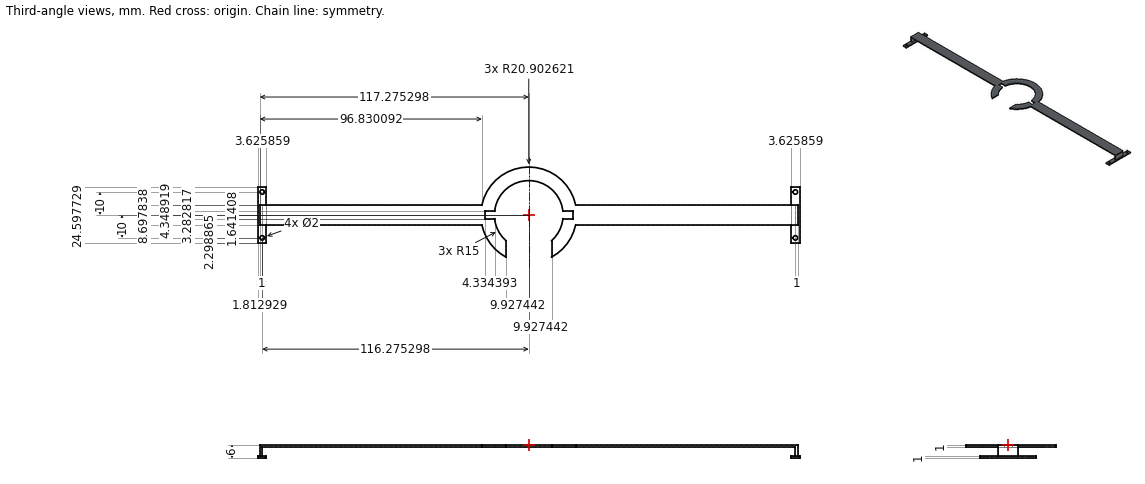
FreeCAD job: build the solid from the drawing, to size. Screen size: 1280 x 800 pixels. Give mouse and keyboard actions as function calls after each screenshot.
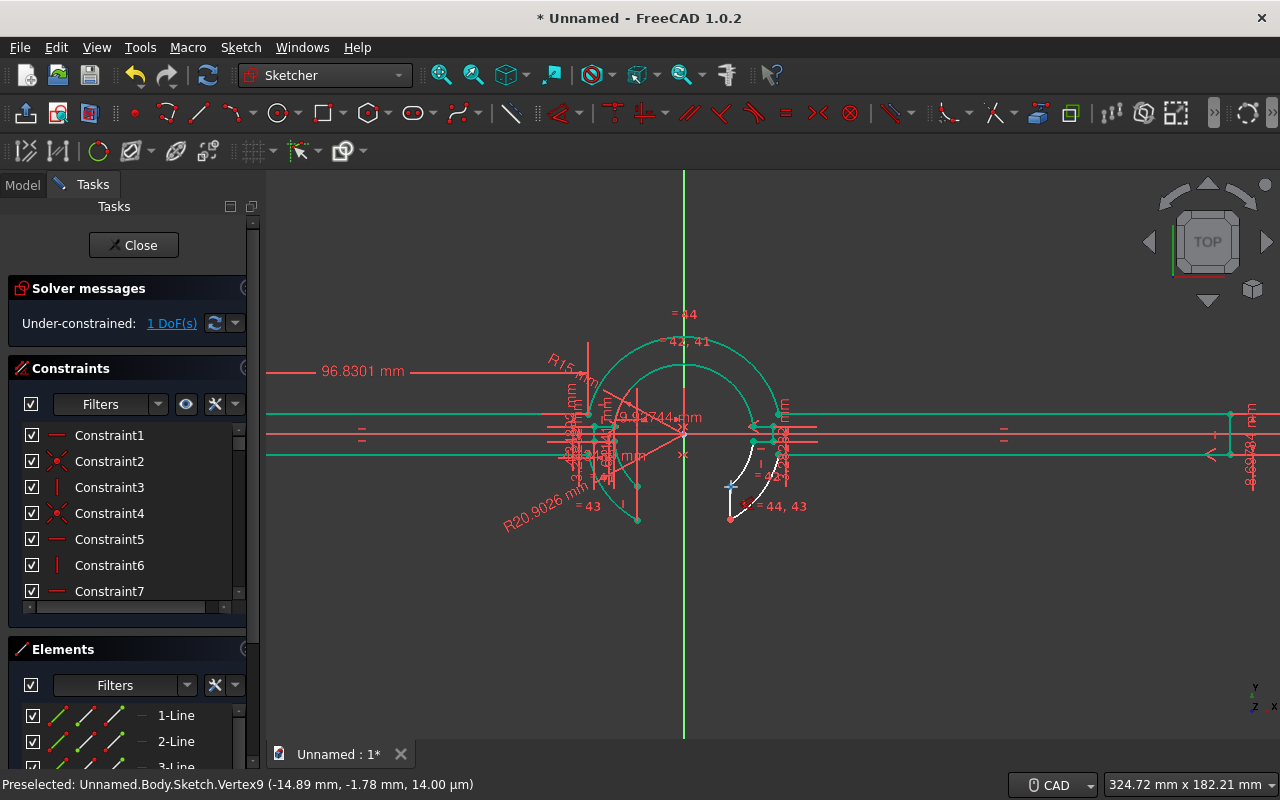
click(730, 486)
click(707, 520)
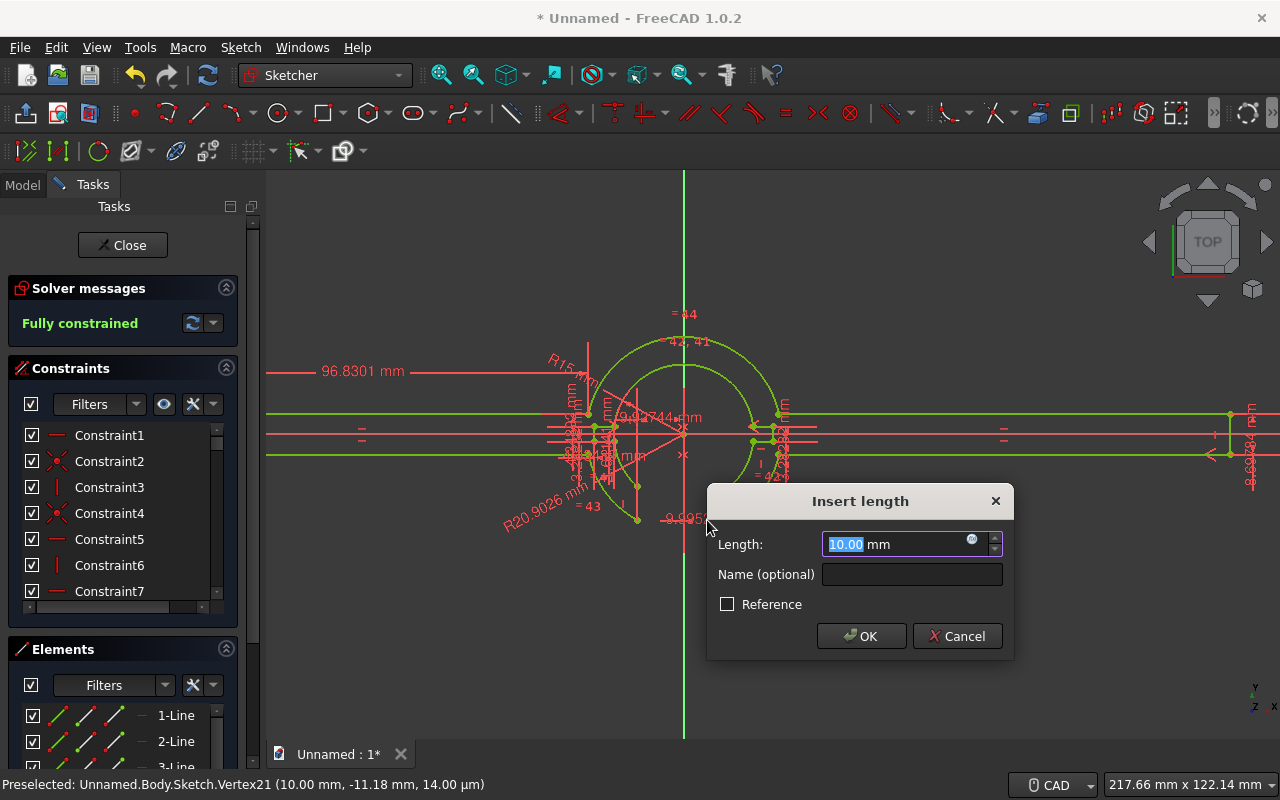
text(9.927442)
key(Return)
key(Escape)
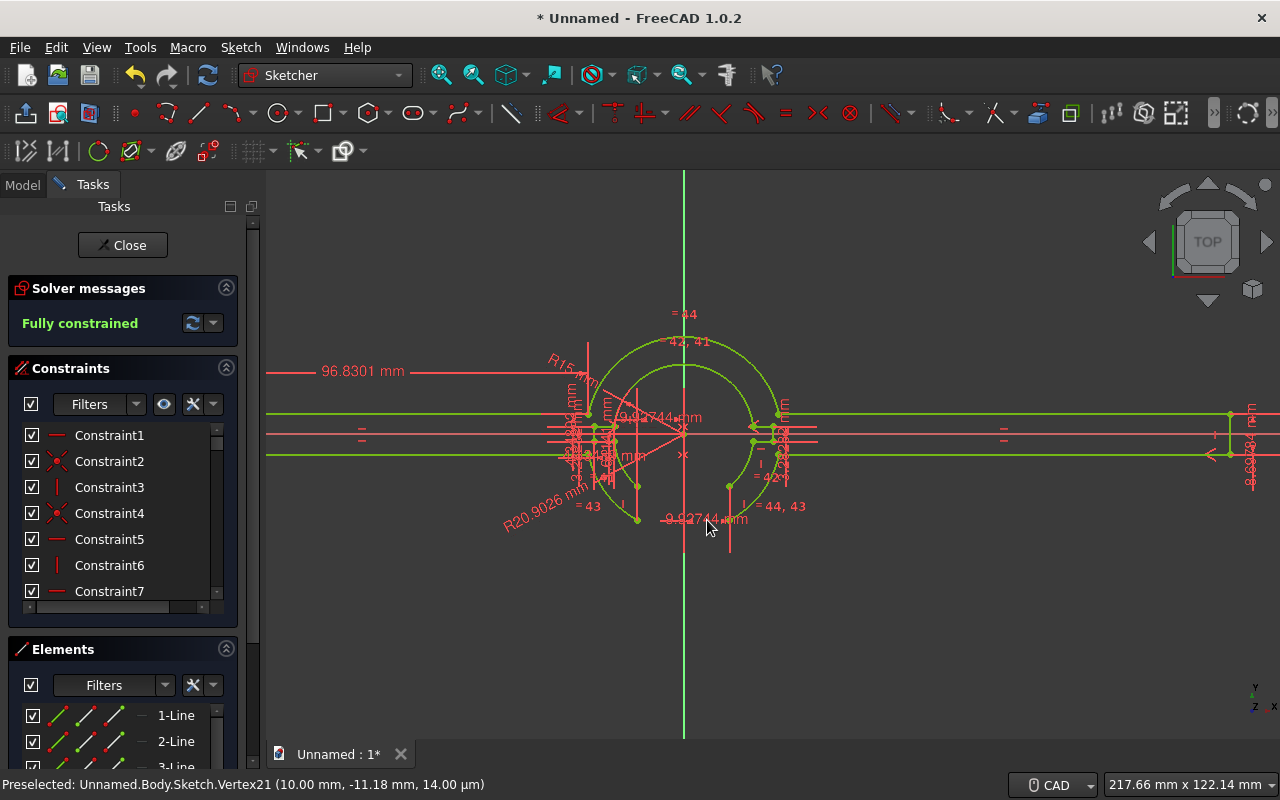
click(123, 245)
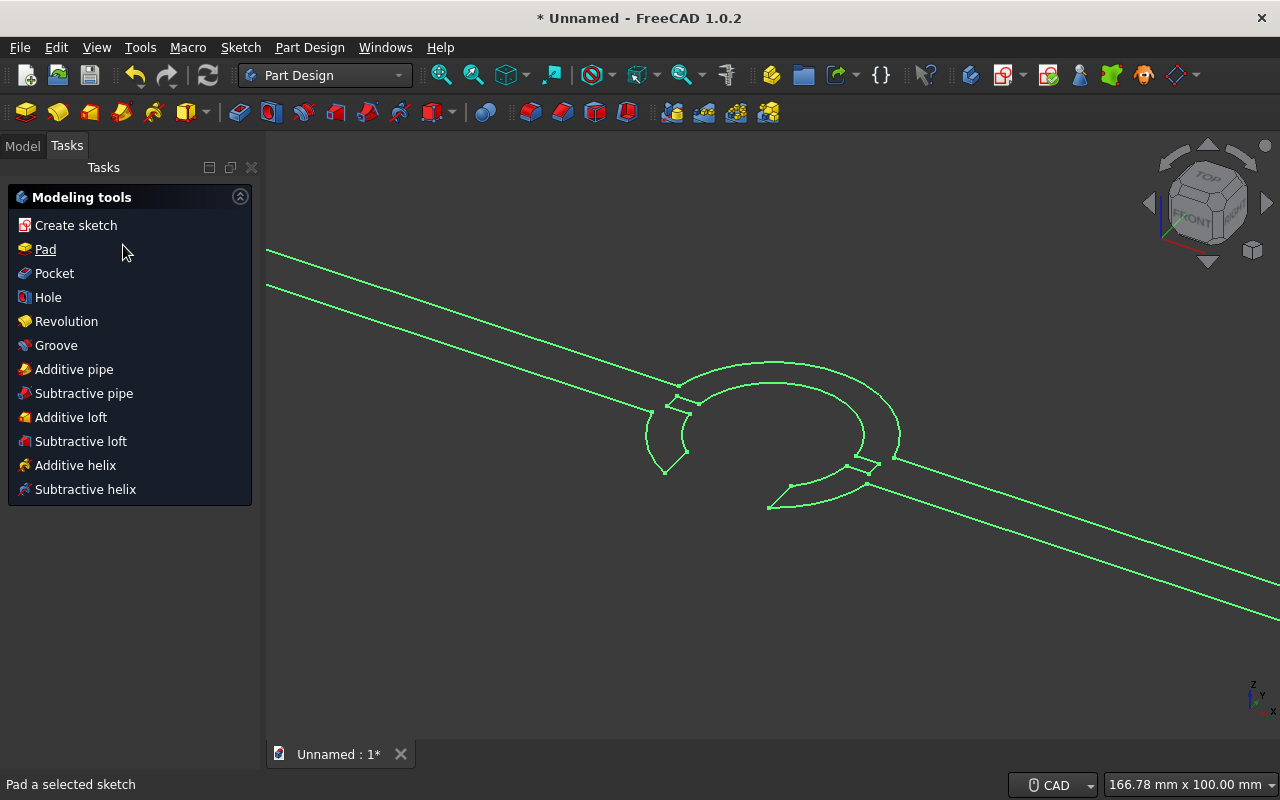
click(26, 112)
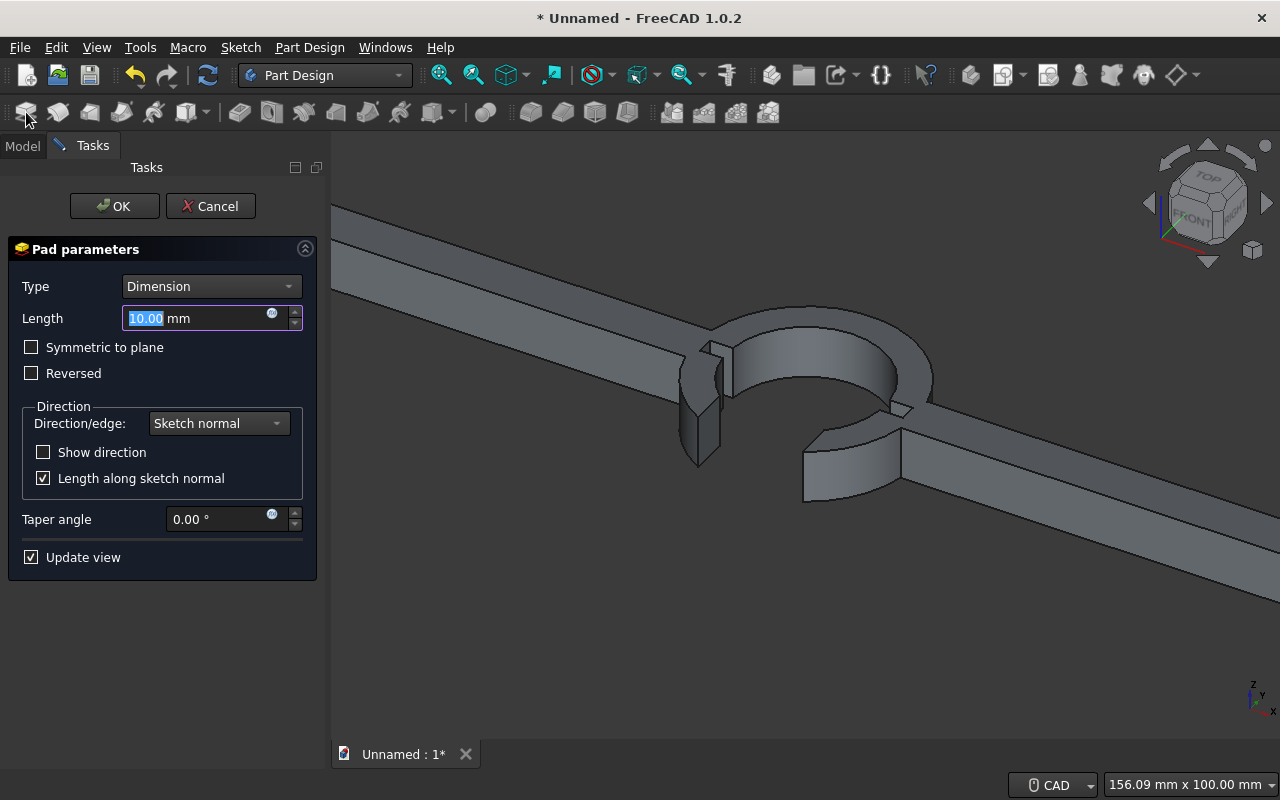
text(1)
key(Tab)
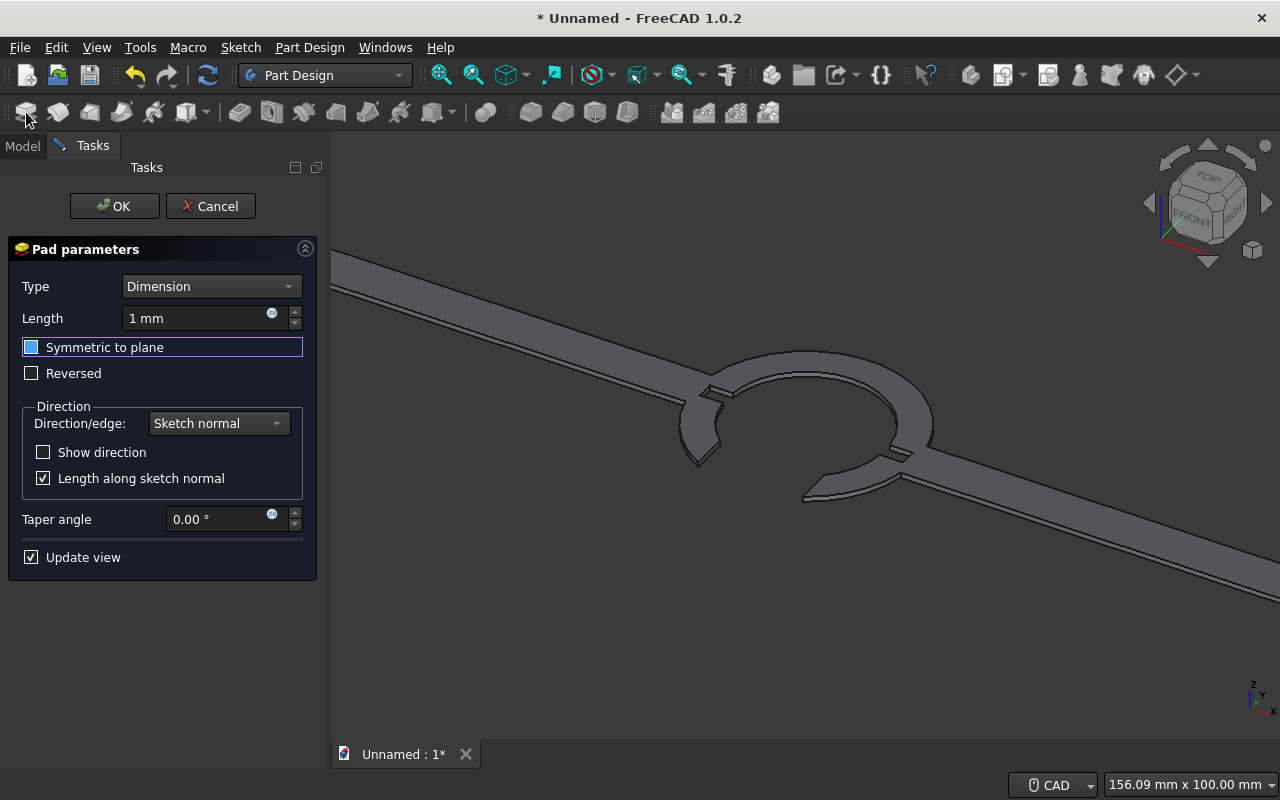
click(30, 373)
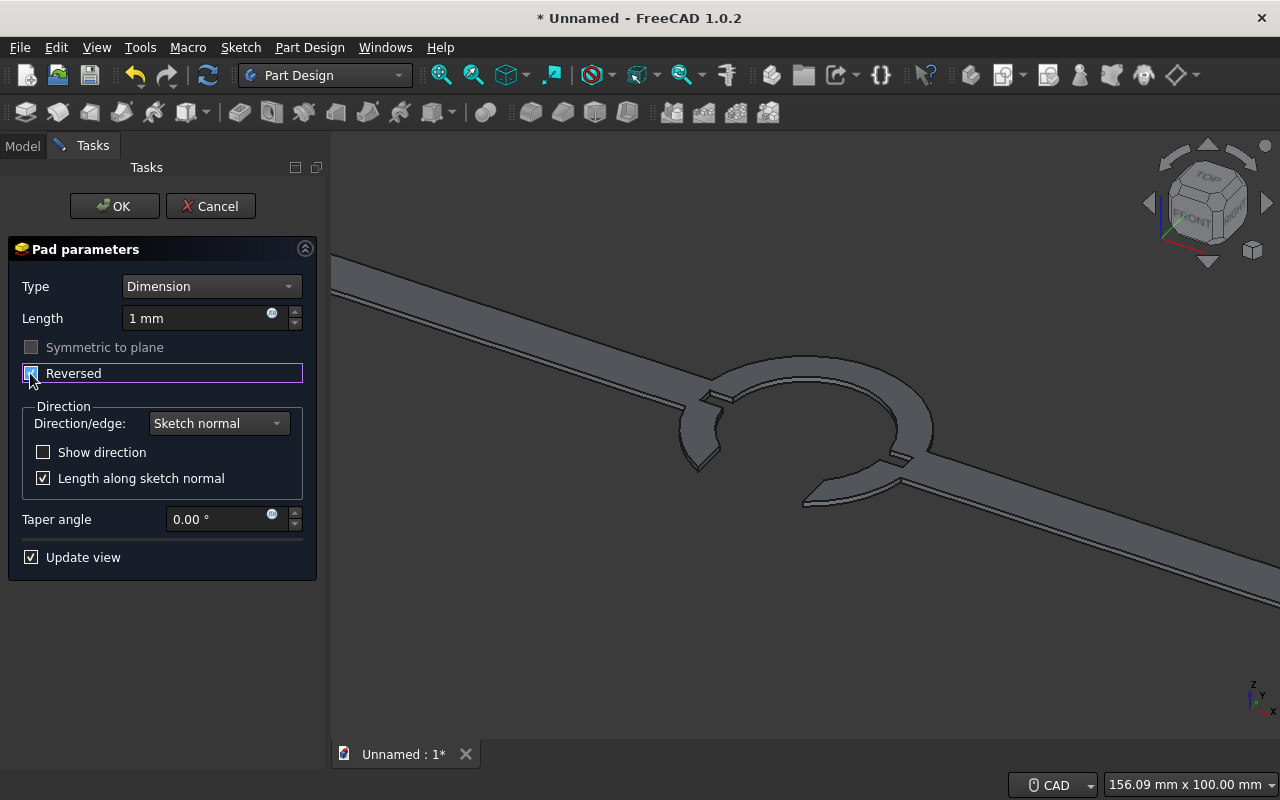
click(115, 206)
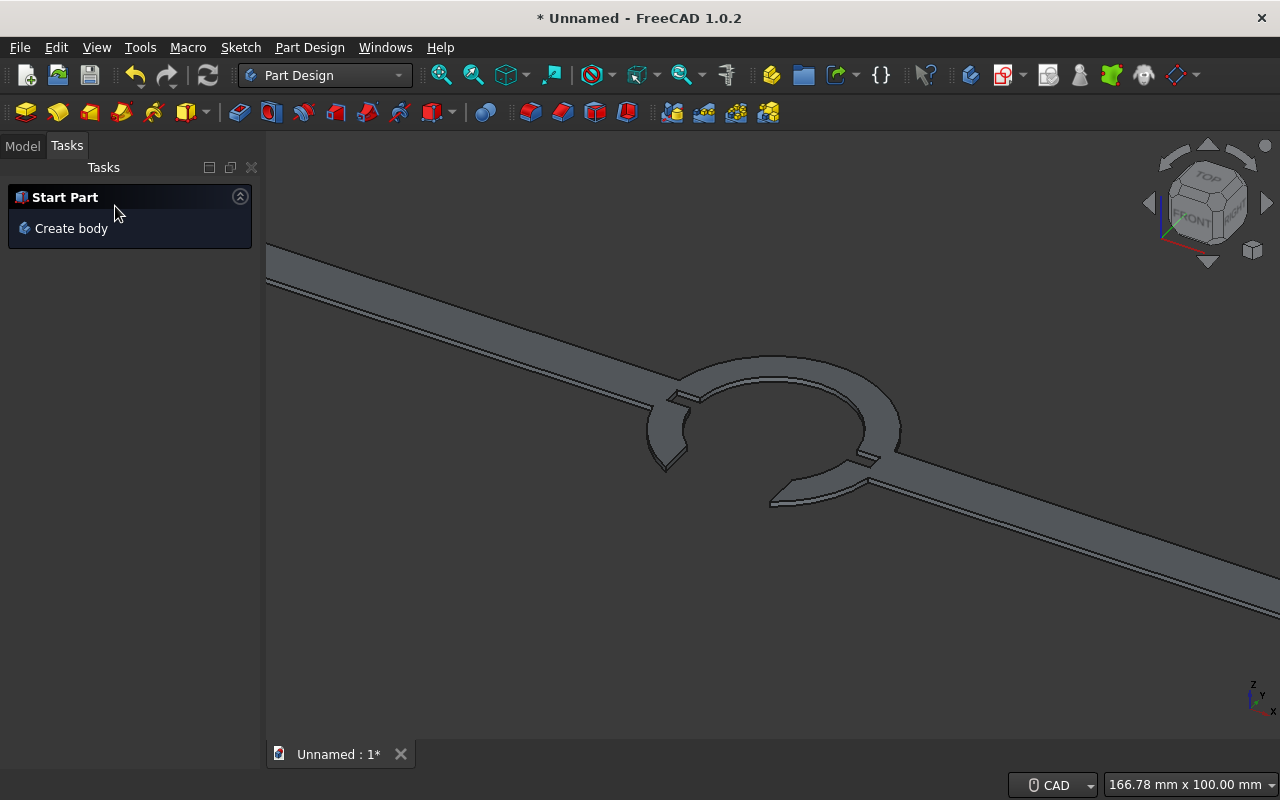
click(442, 76)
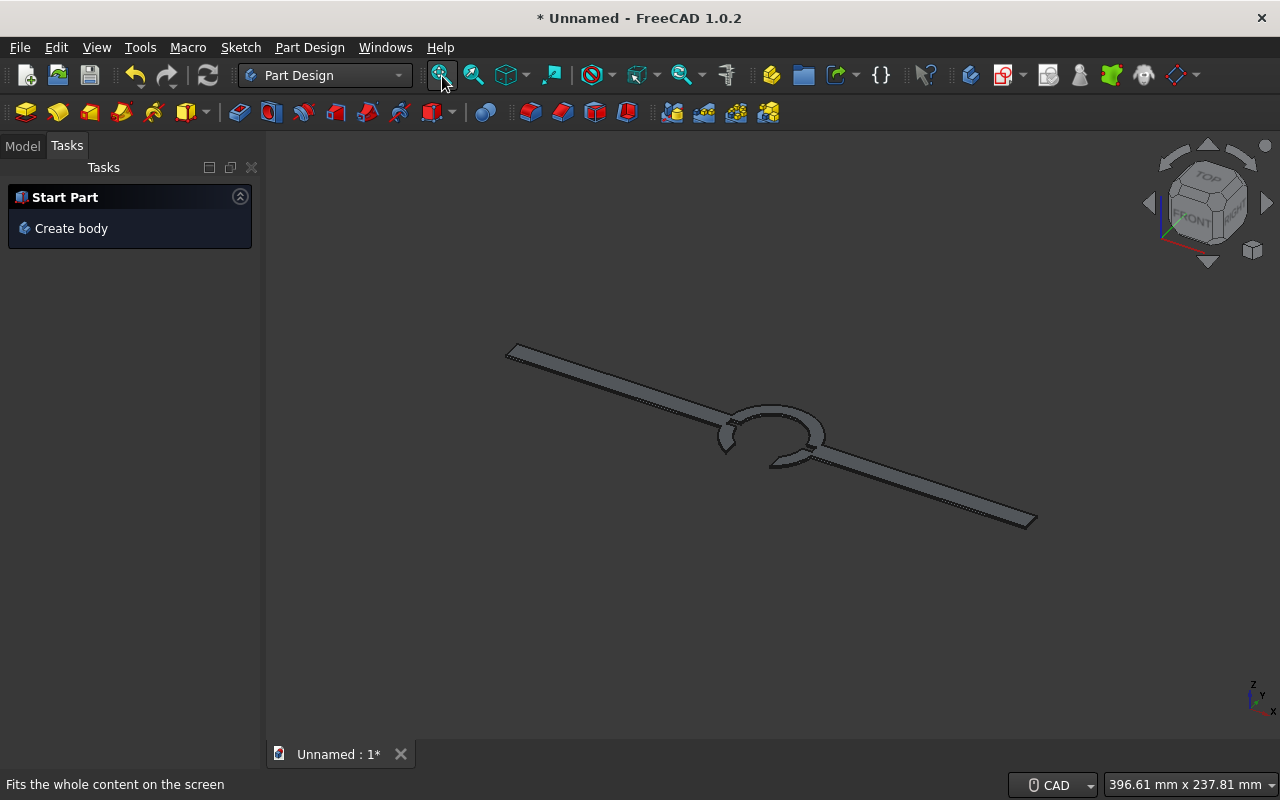
click(921, 482)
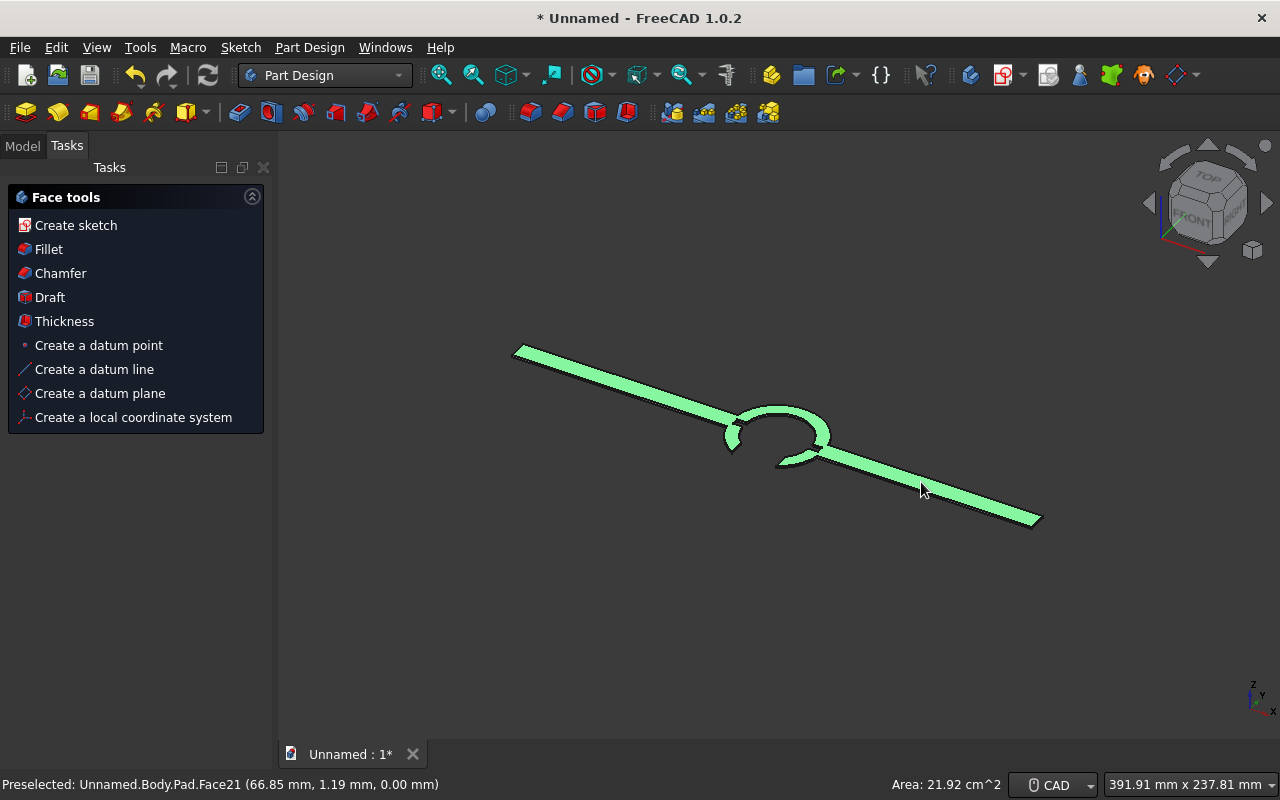
click(1004, 76)